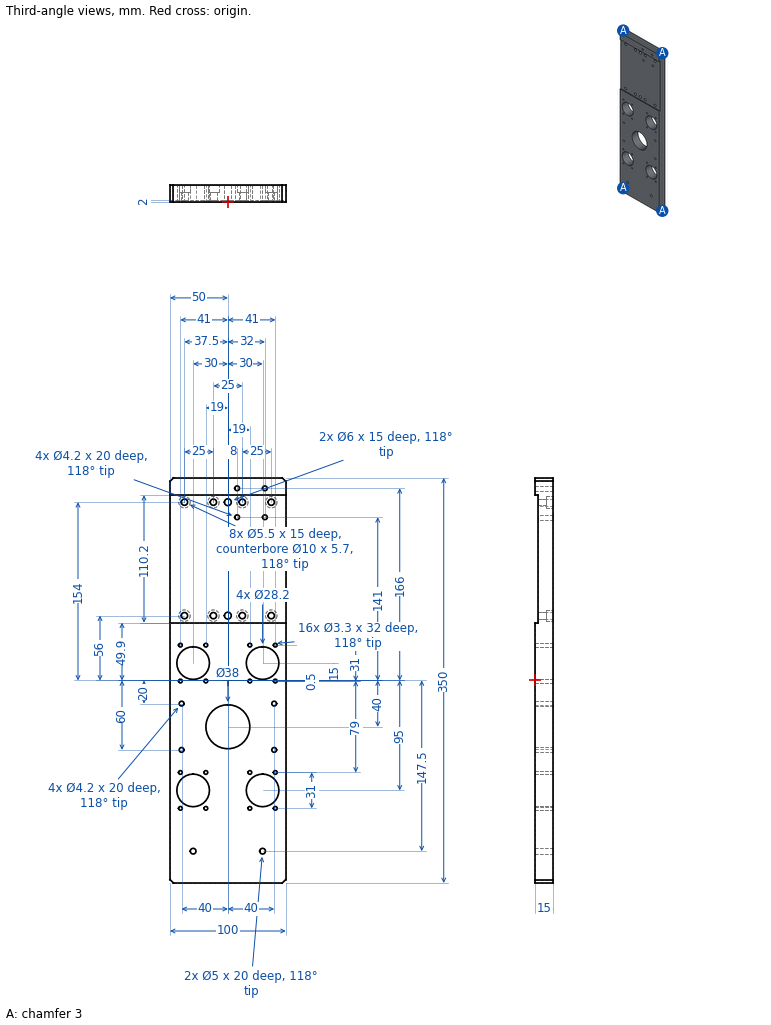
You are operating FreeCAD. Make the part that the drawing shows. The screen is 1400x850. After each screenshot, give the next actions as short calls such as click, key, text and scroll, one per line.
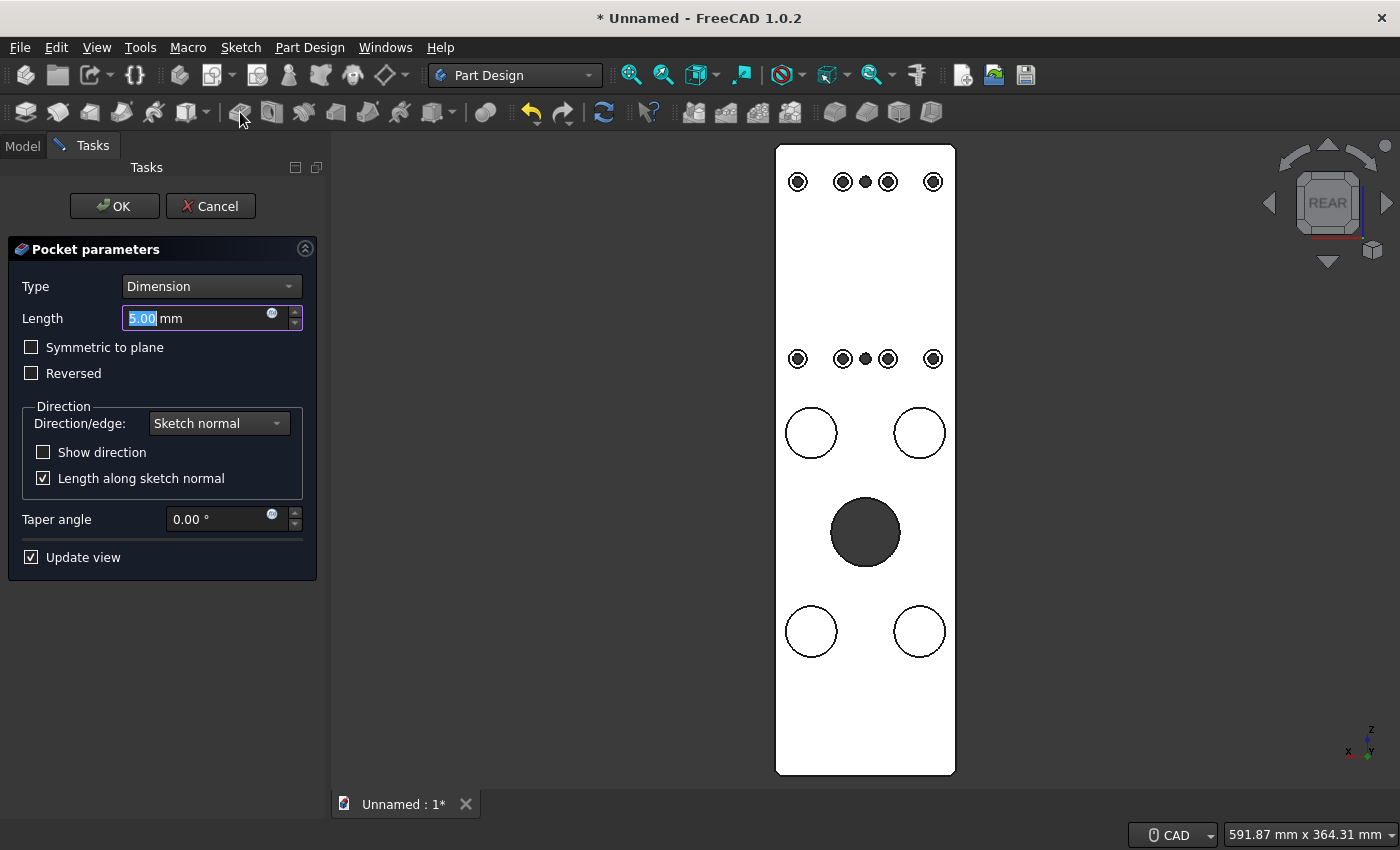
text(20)
key(Tab)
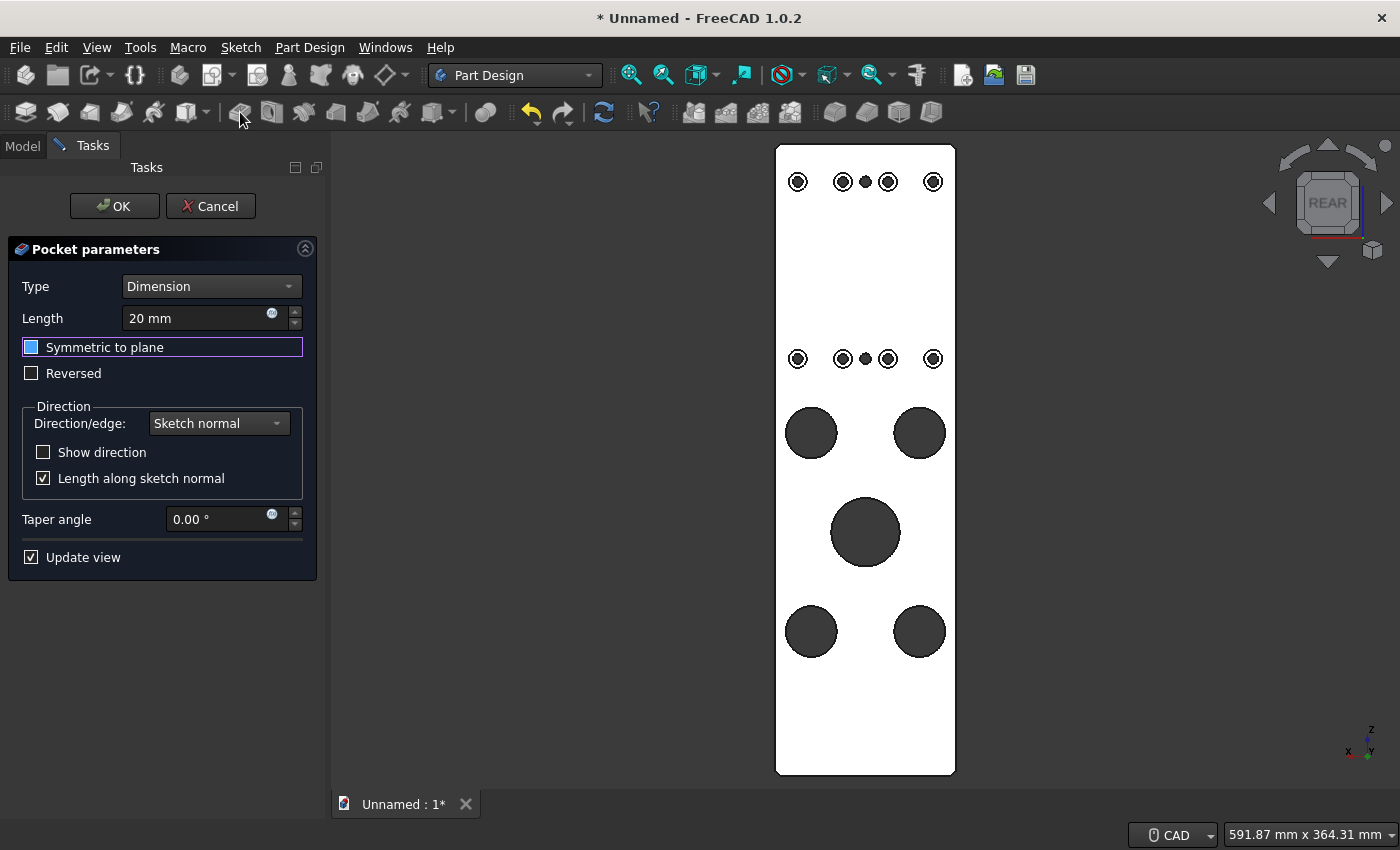
click(115, 206)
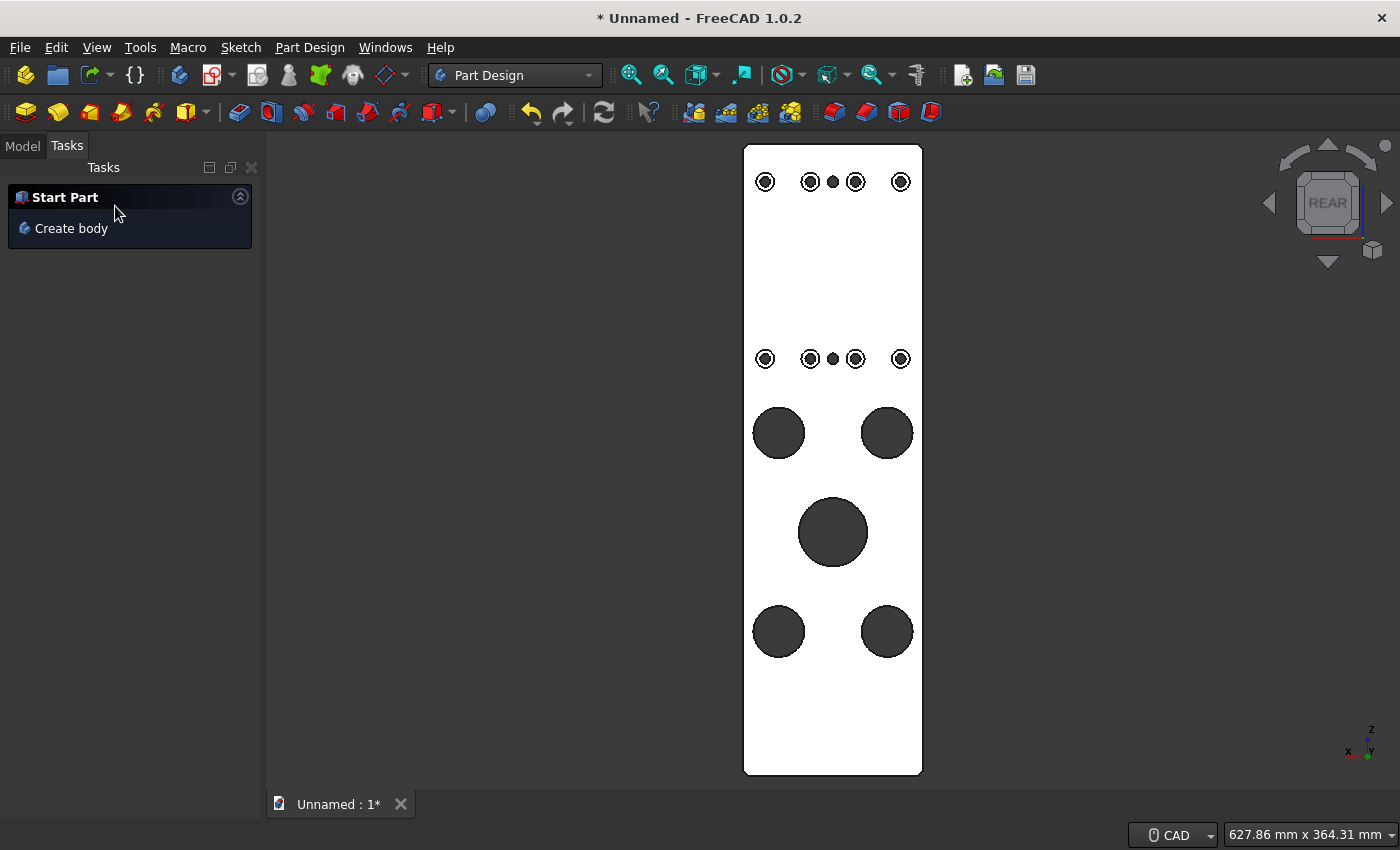
click(833, 278)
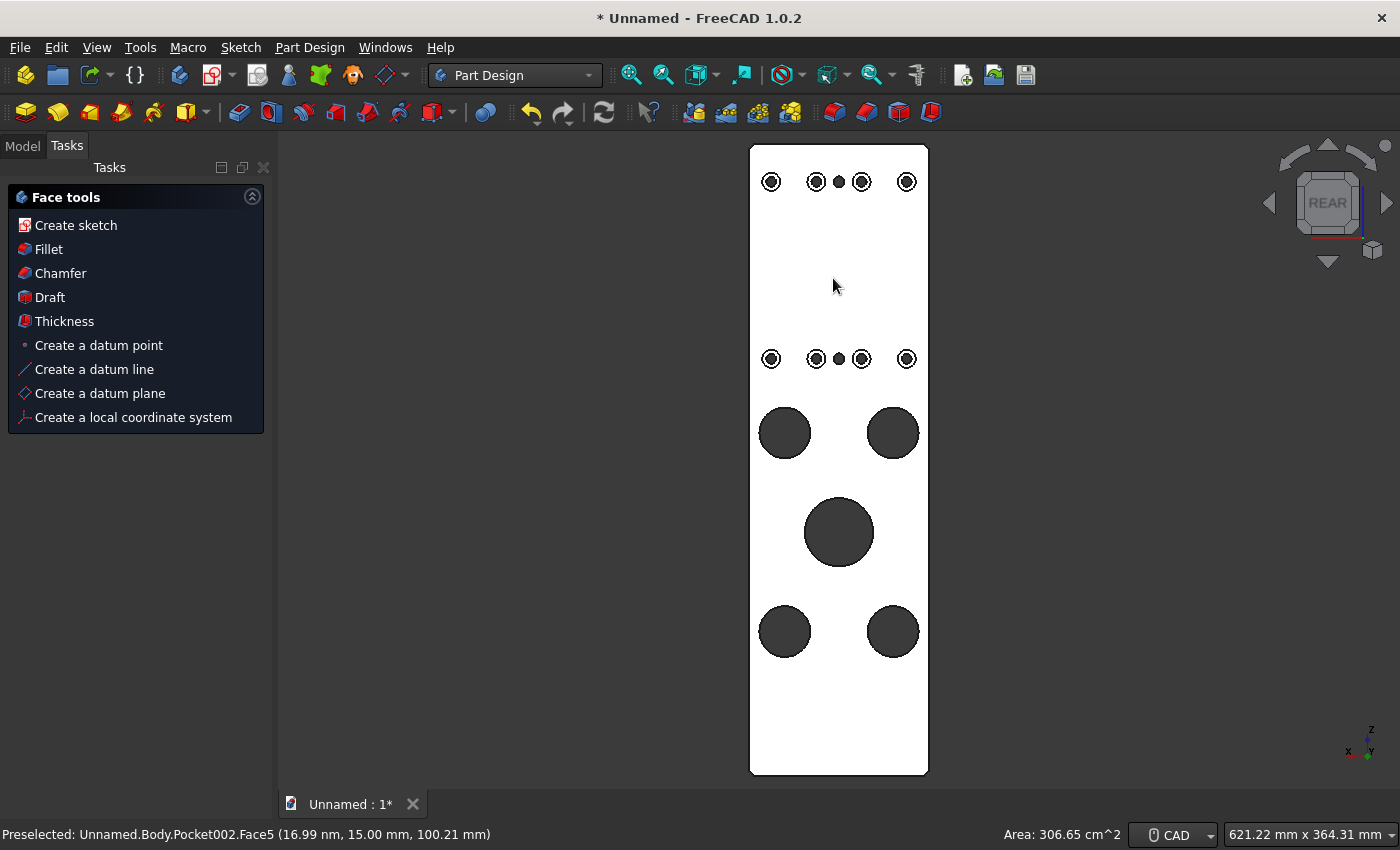
click(212, 76)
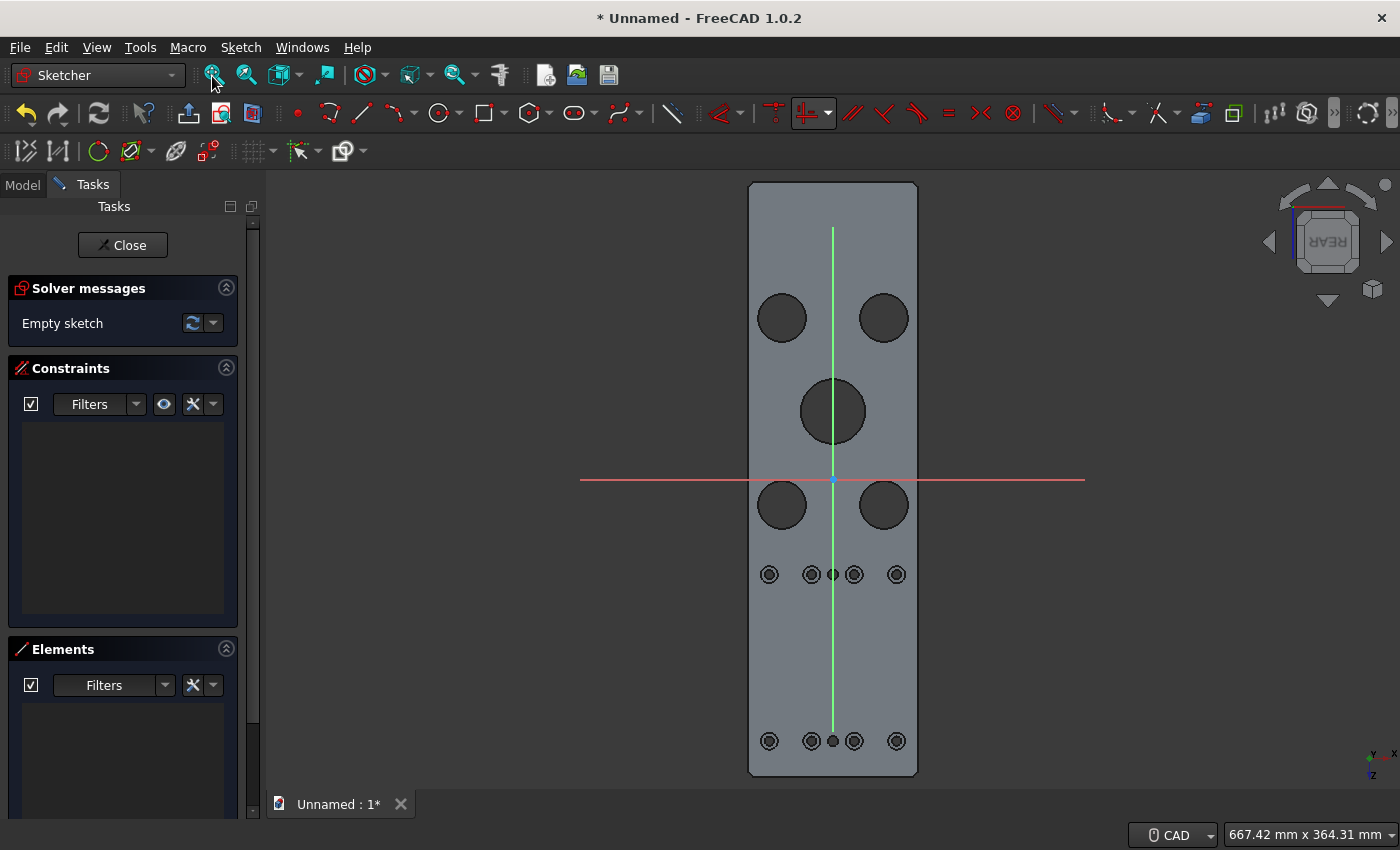
scroll(972, 198, up, 2)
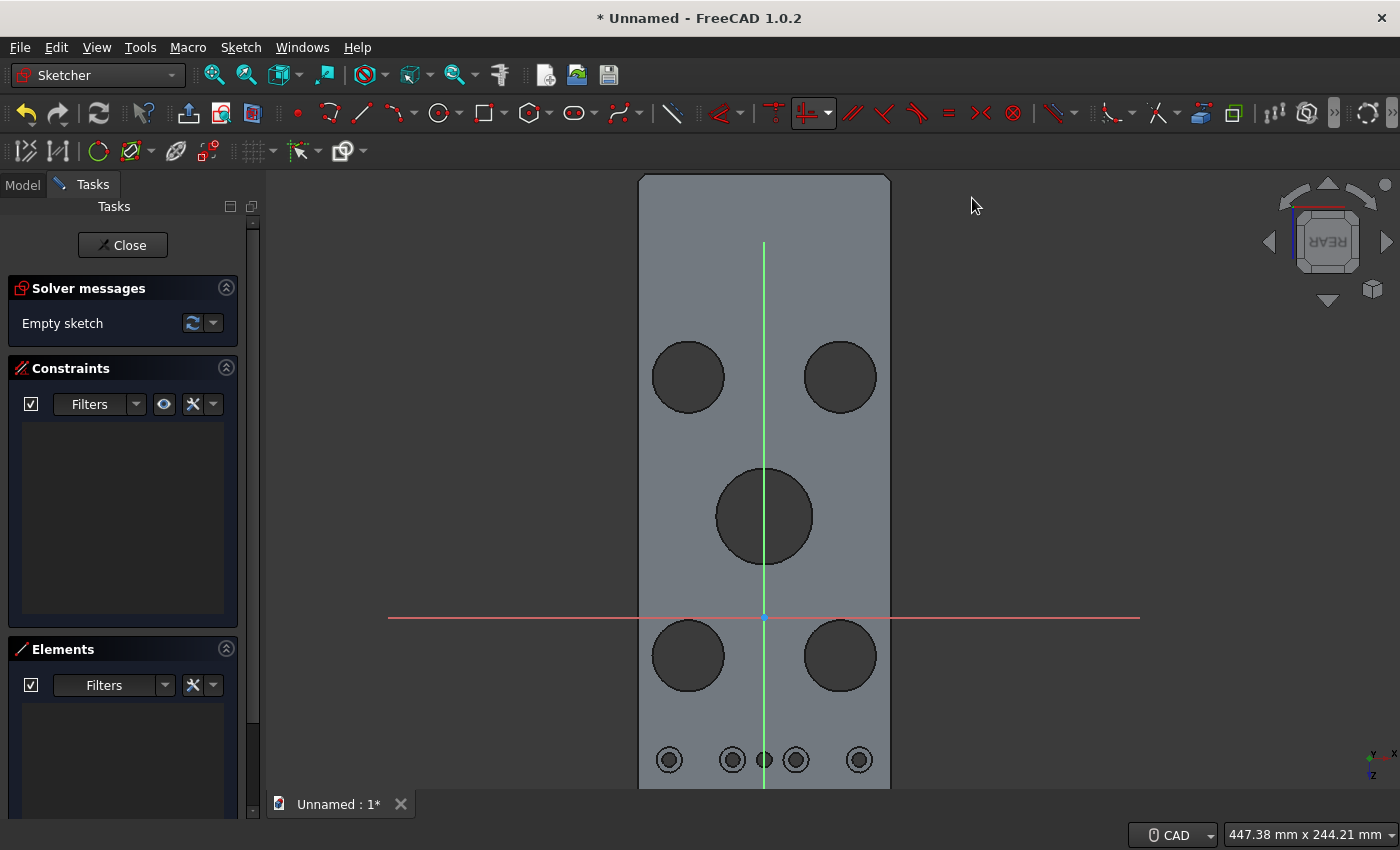
click(440, 114)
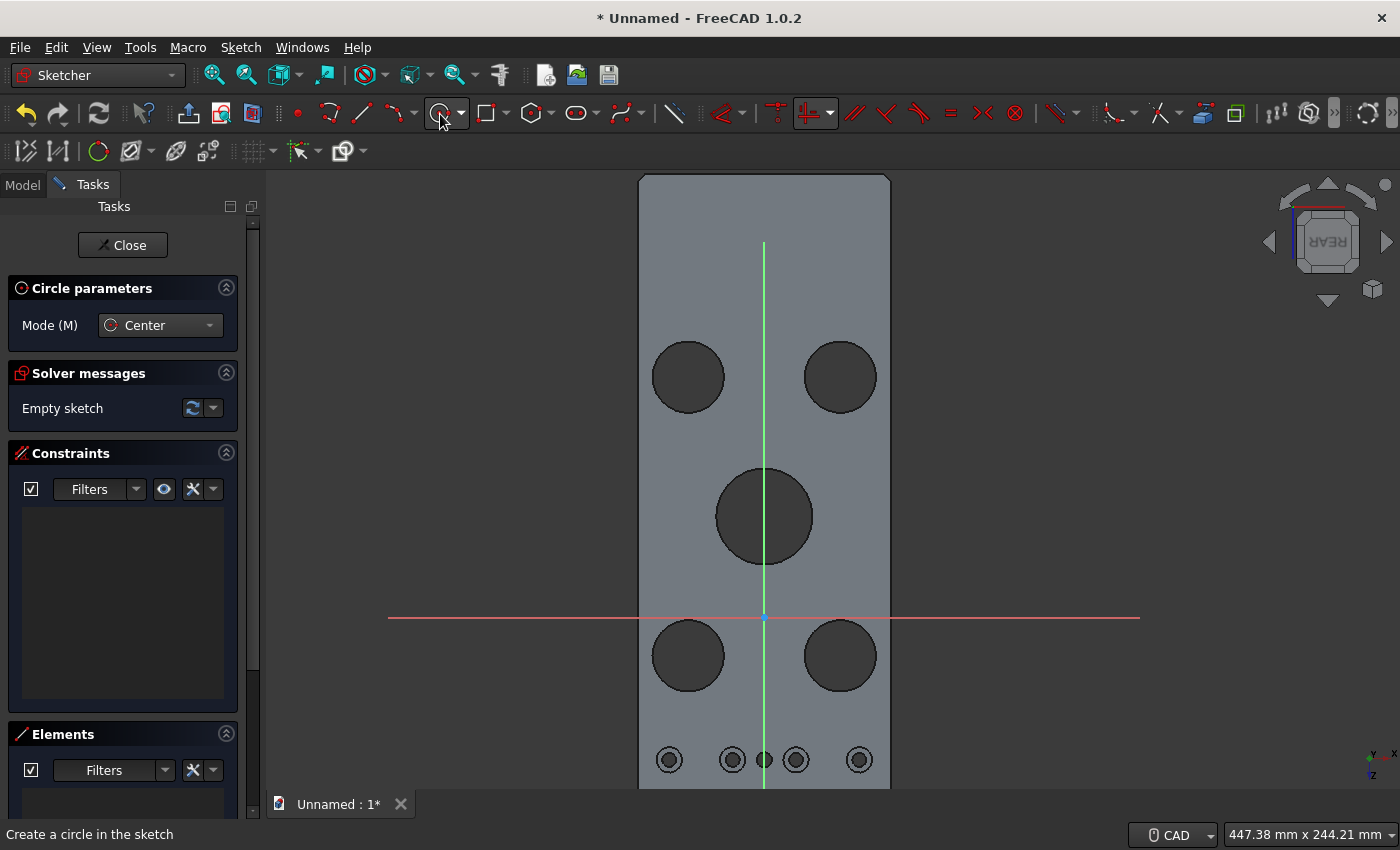
scroll(840, 244, up, 7)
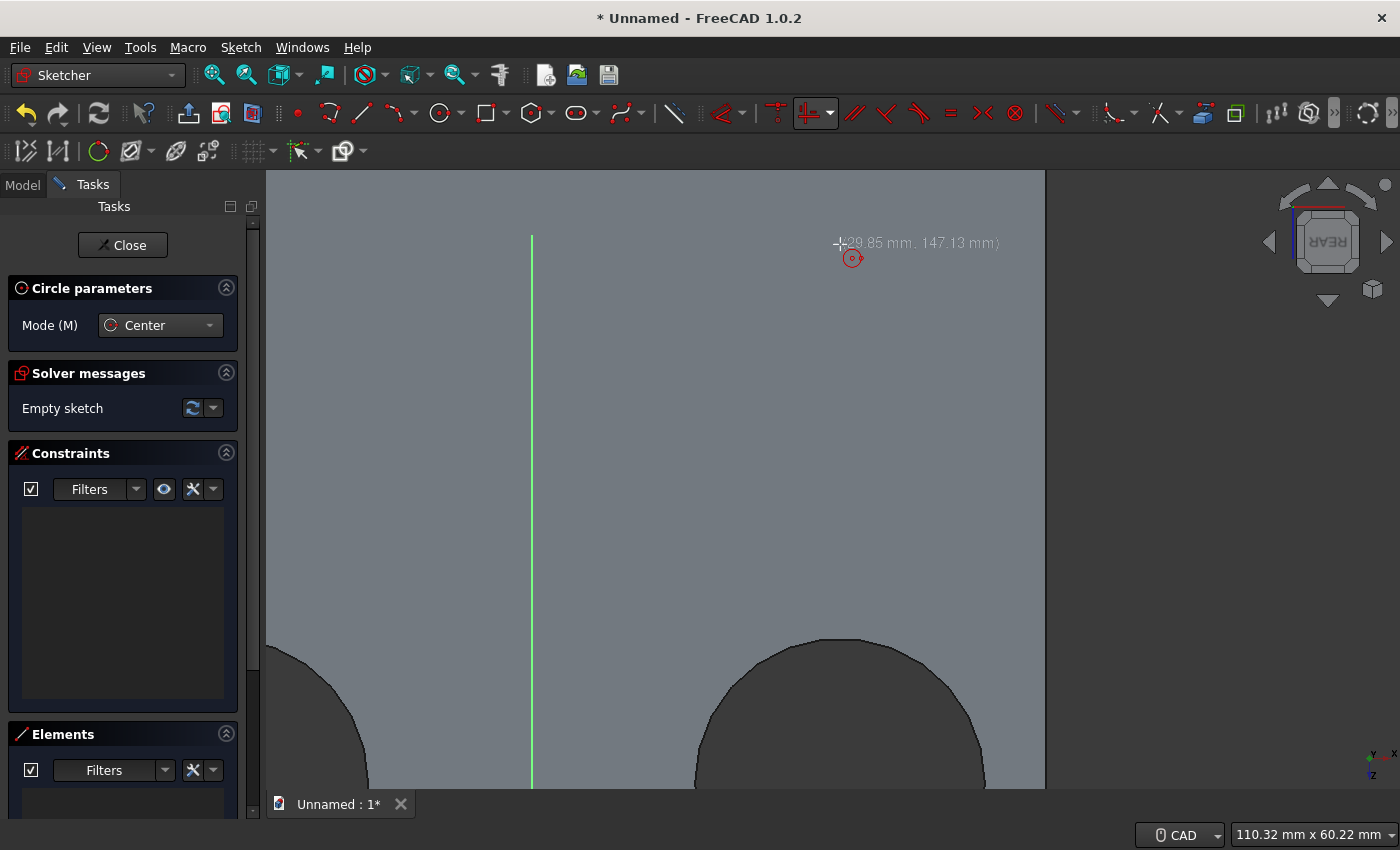
scroll(841, 313, down, 7)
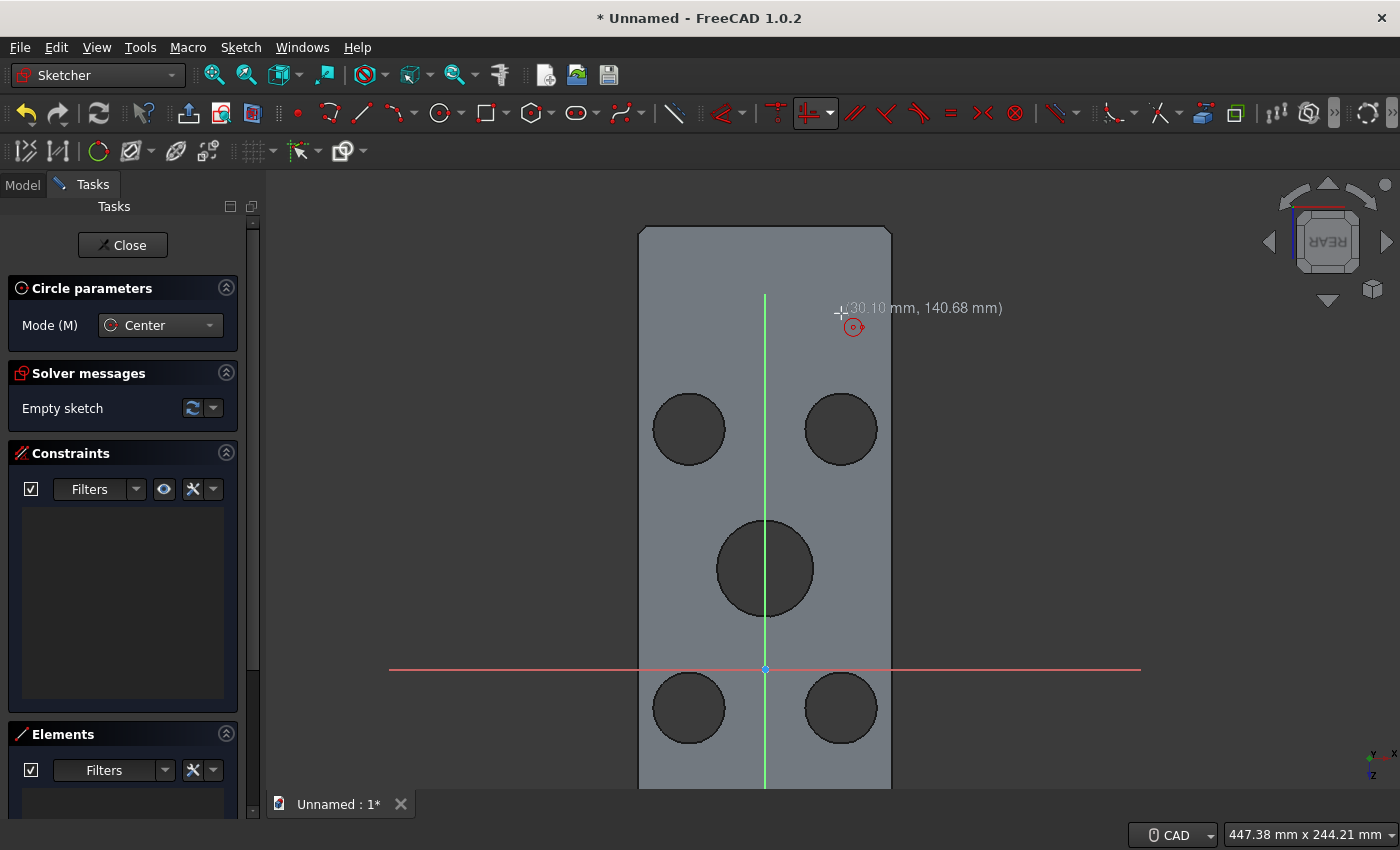
click(841, 296)